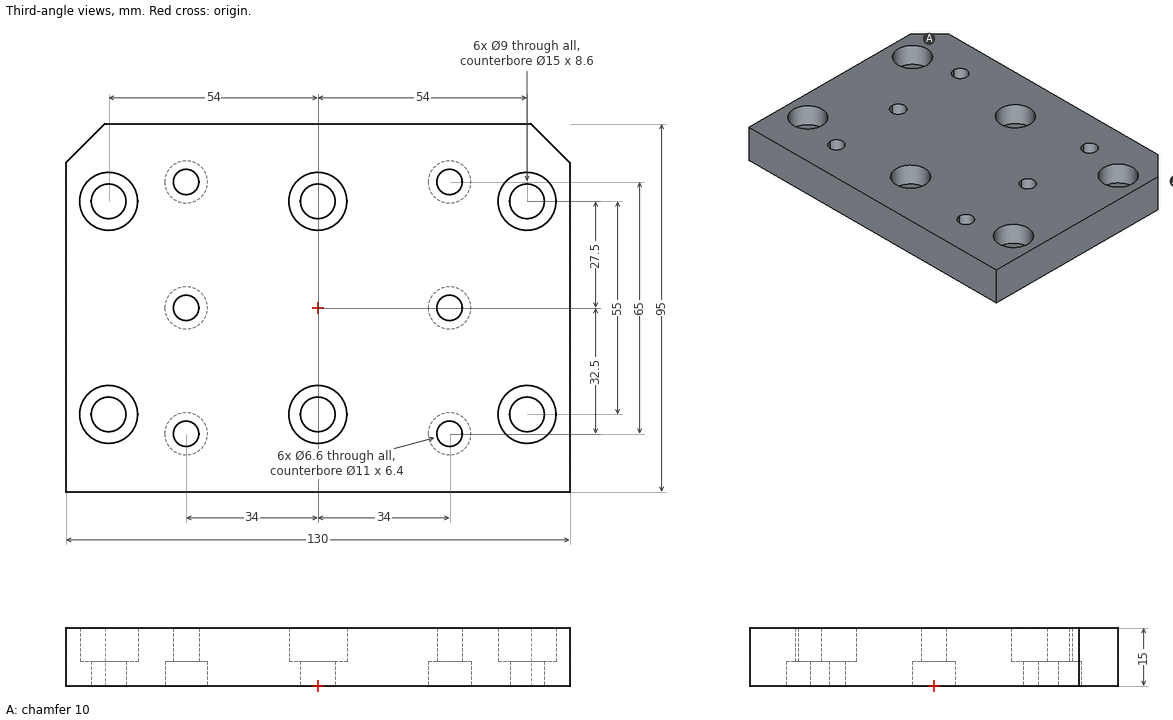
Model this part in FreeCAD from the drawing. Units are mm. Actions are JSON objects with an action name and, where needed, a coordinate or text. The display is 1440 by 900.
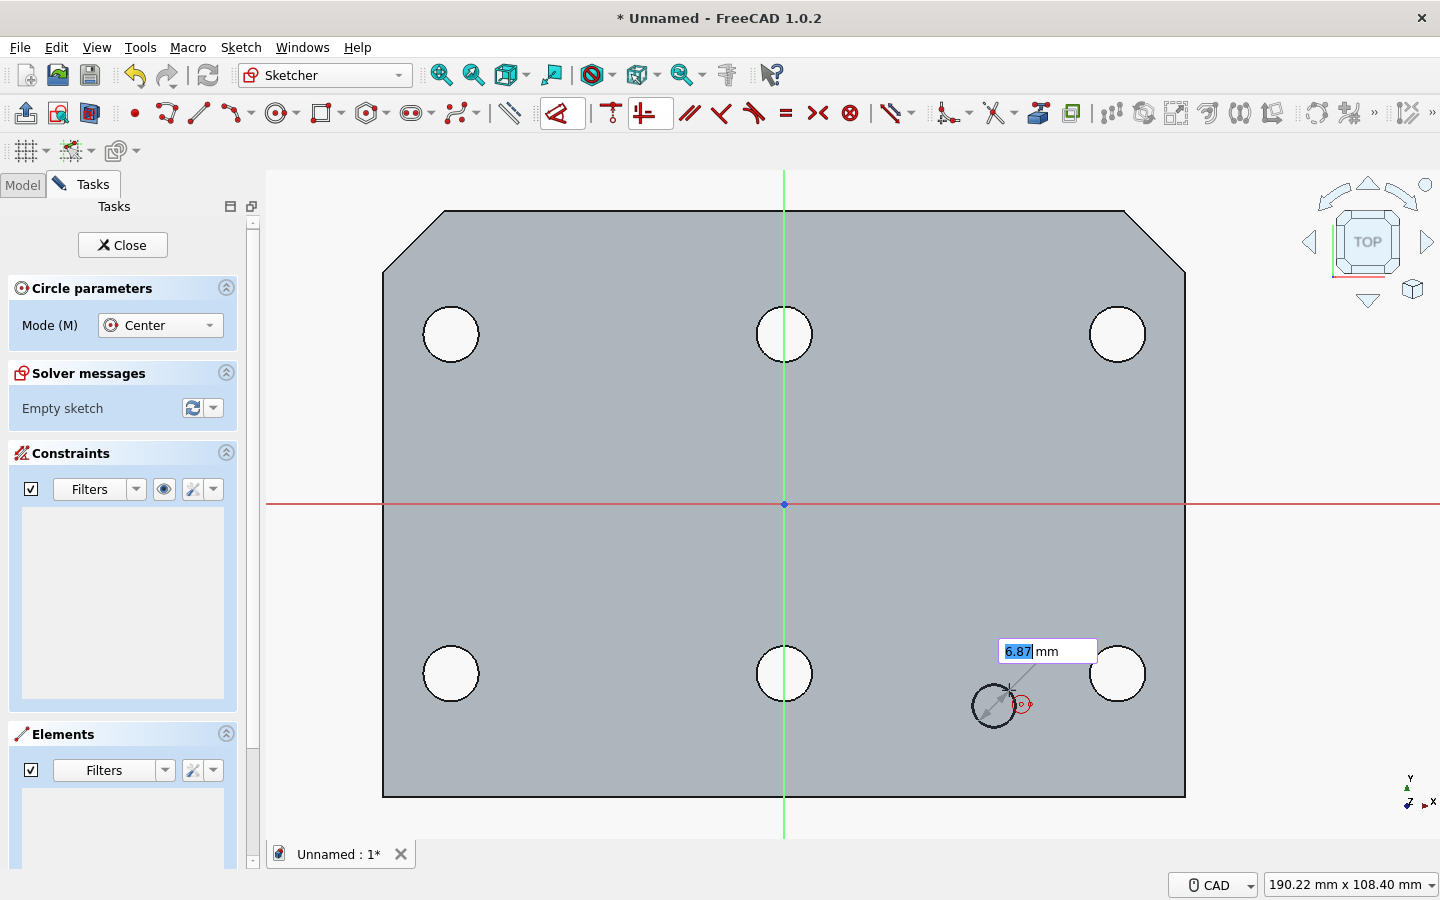
{"action": "type", "text": "6.6"}
{"action": "key", "text": "Return"}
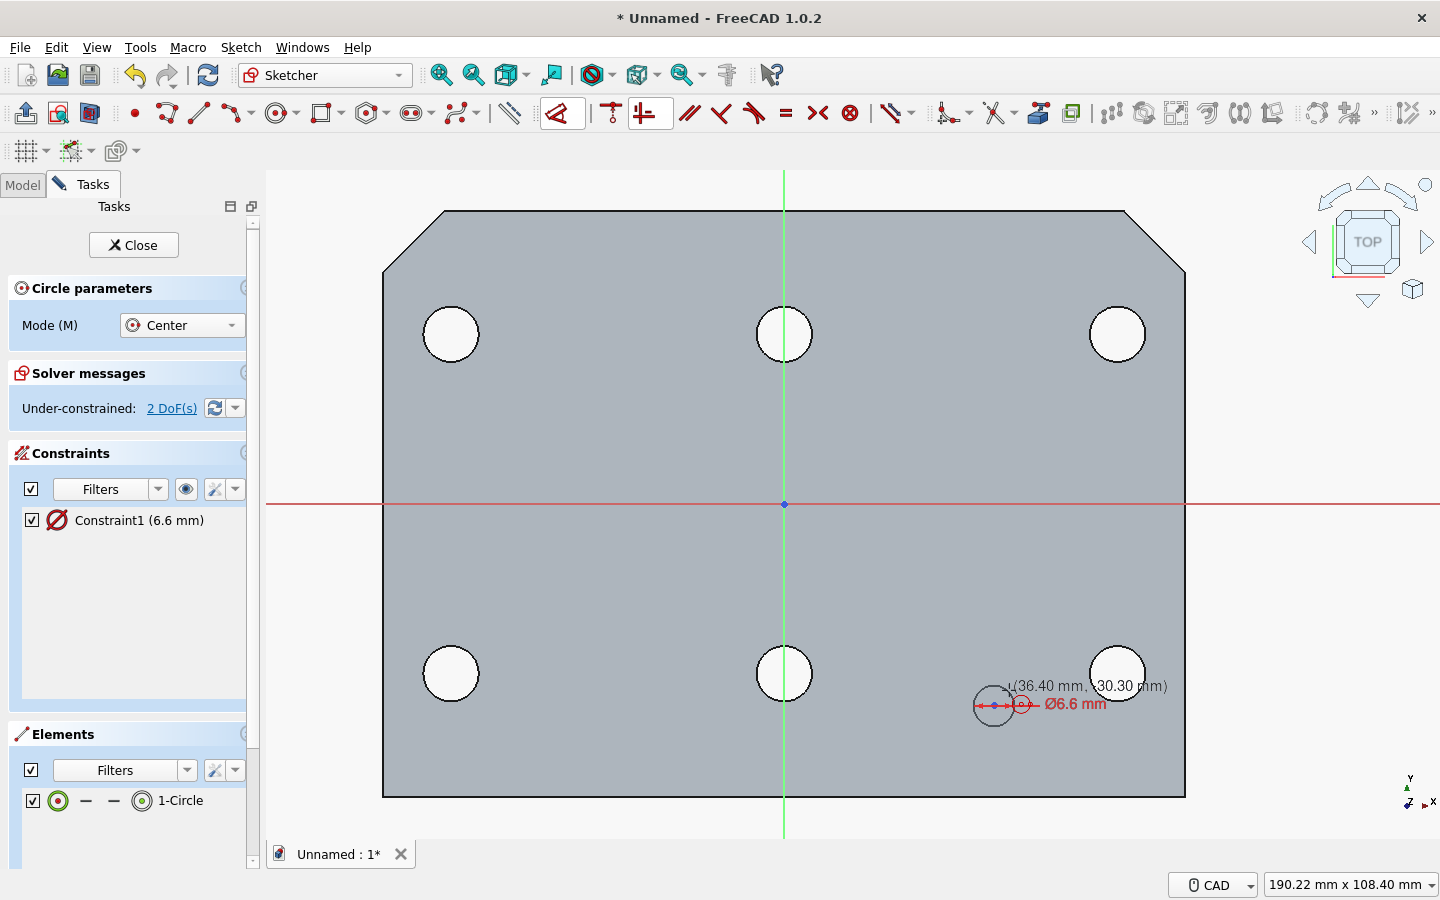
{"action": "left_click", "coordinate": [994, 504]}
{"action": "mouse_move", "coordinate": [1009, 490]}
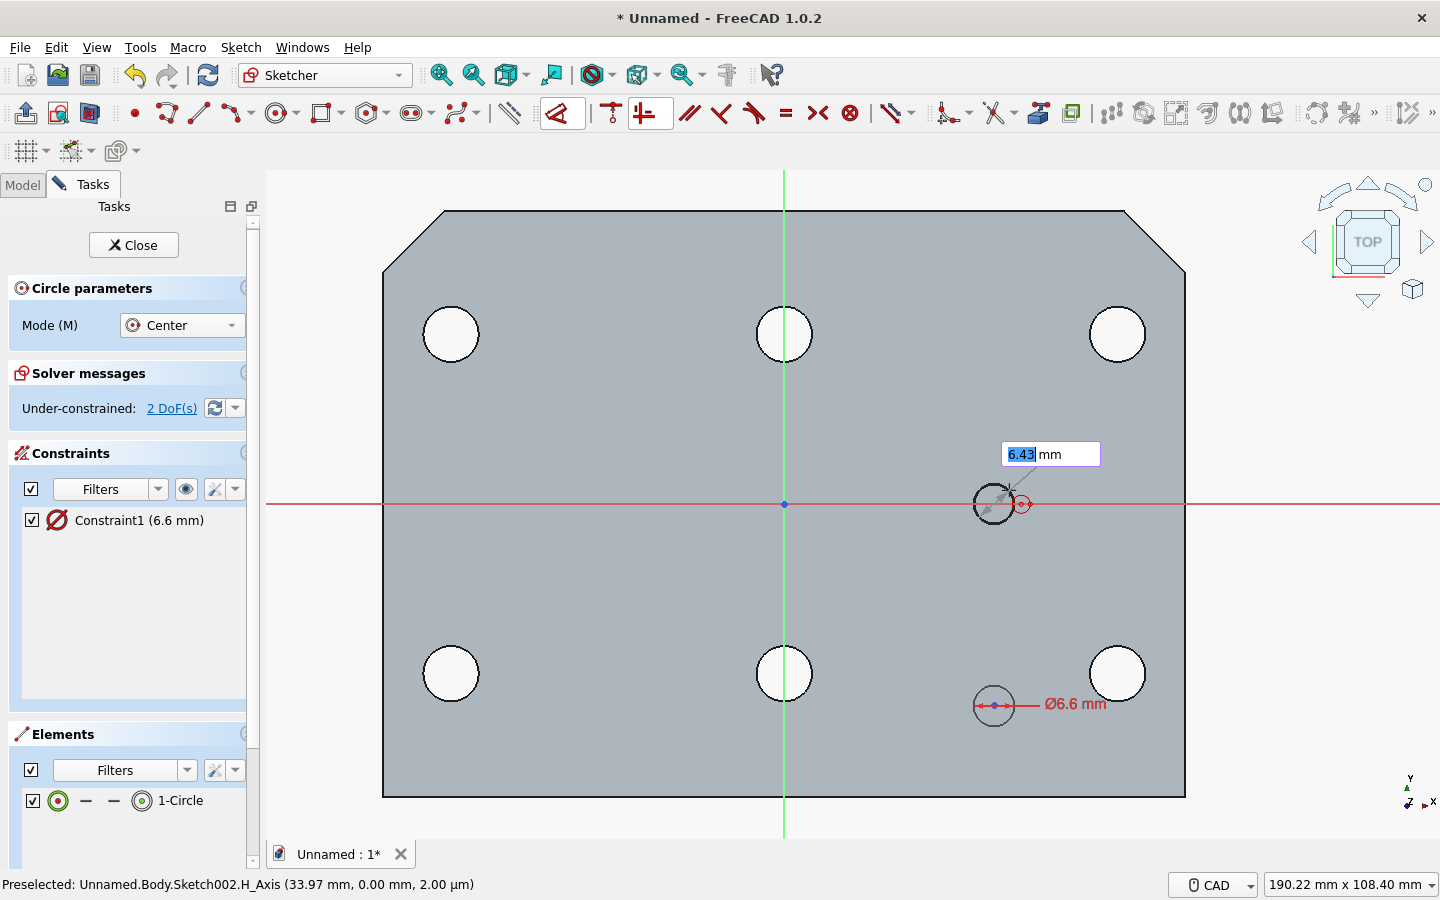
{"action": "type", "text": "6.6"}
{"action": "key", "text": "Return"}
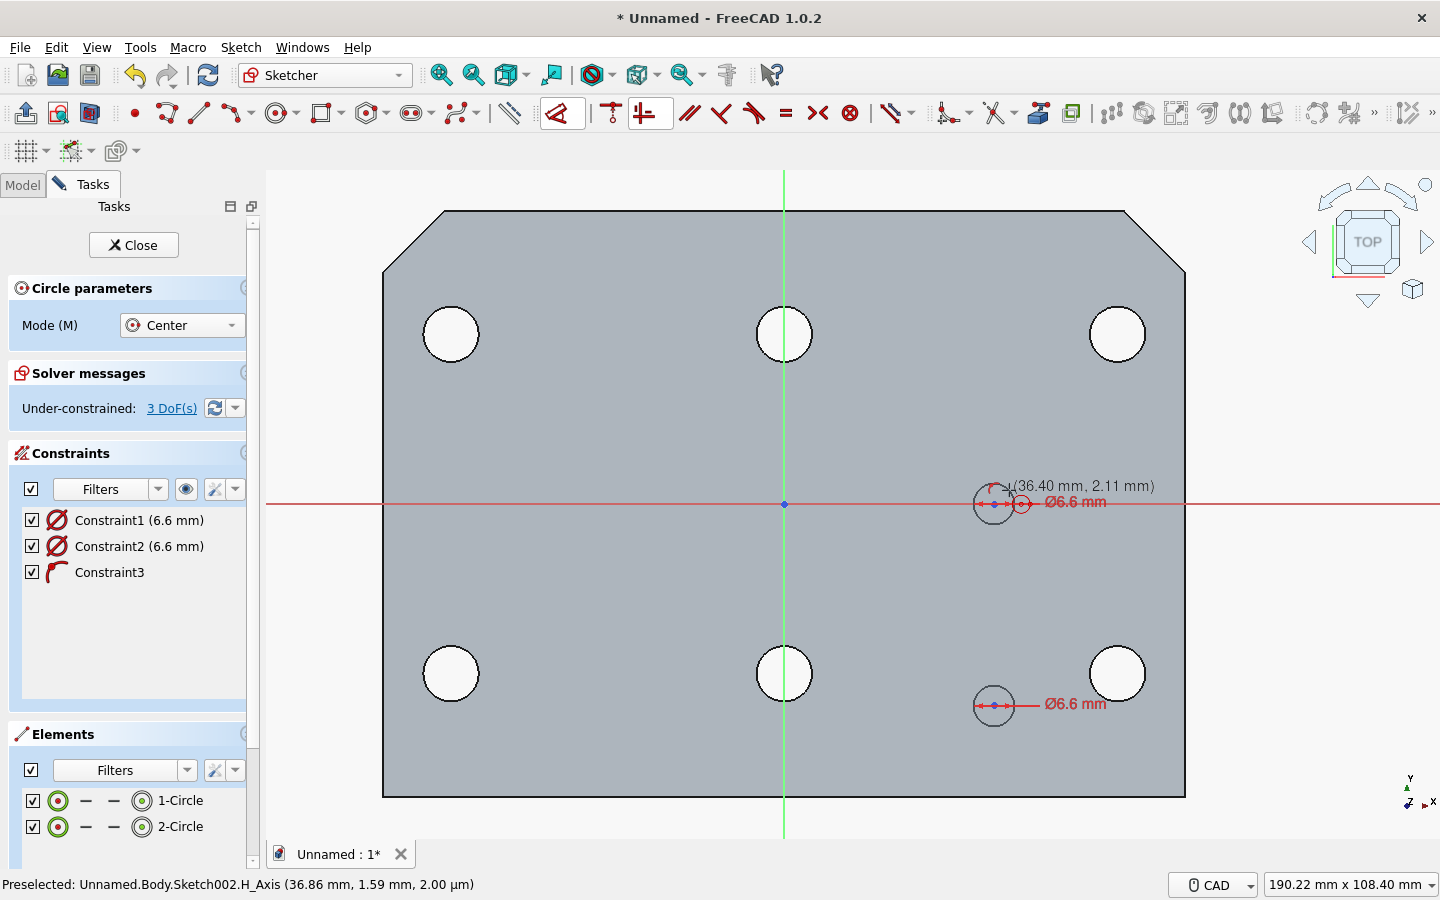
{"action": "left_click", "coordinate": [994, 303]}
{"action": "mouse_move", "coordinate": [1009, 289]}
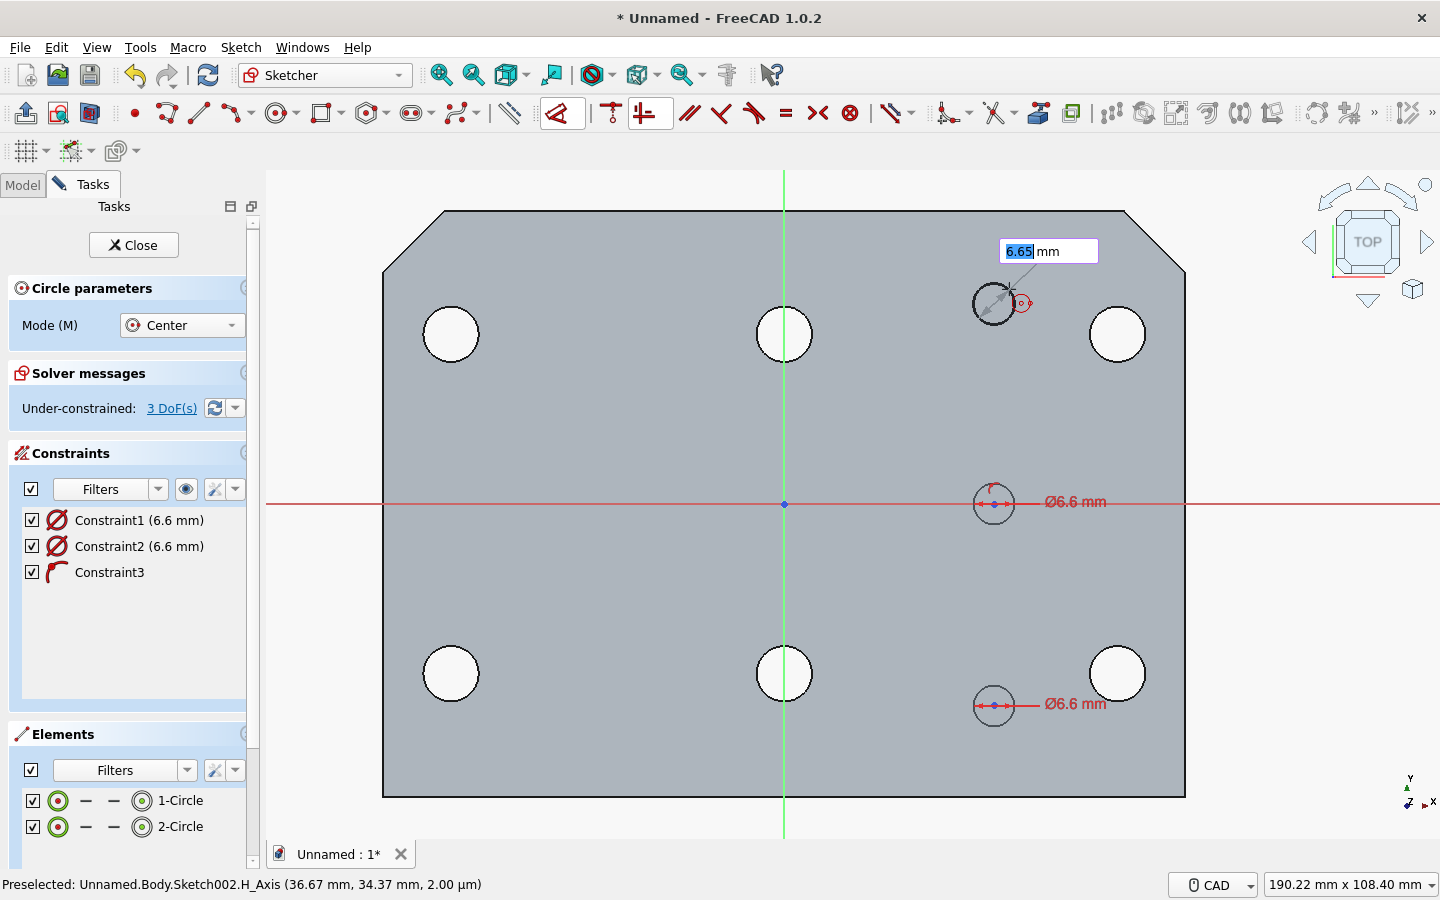
{"action": "type", "text": "6.6"}
{"action": "key", "text": "Return"}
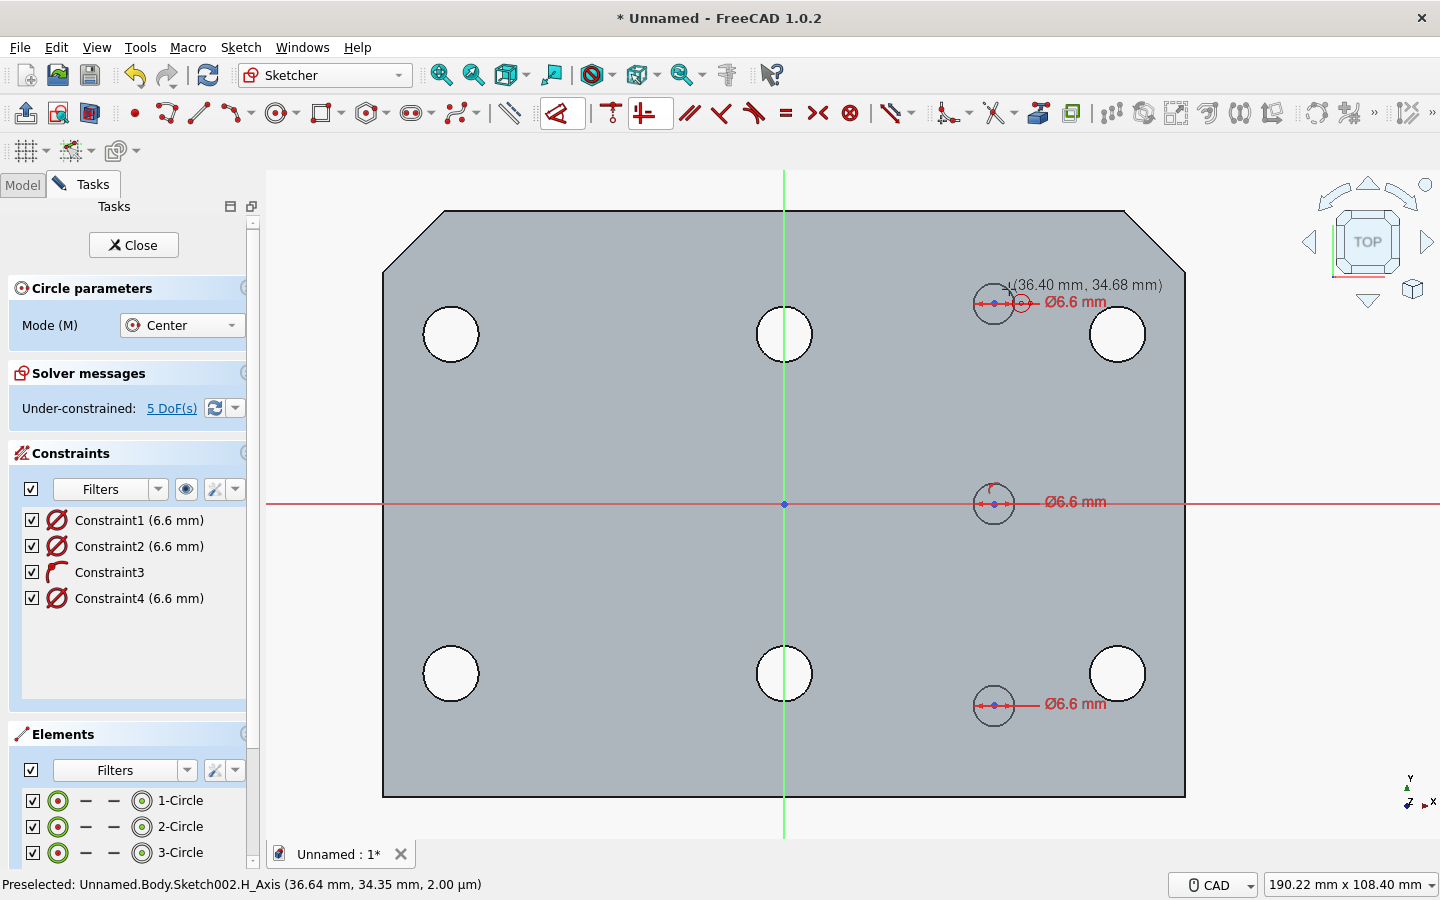
{"action": "left_click", "coordinate": [574, 705]}
{"action": "mouse_move", "coordinate": [589, 690]}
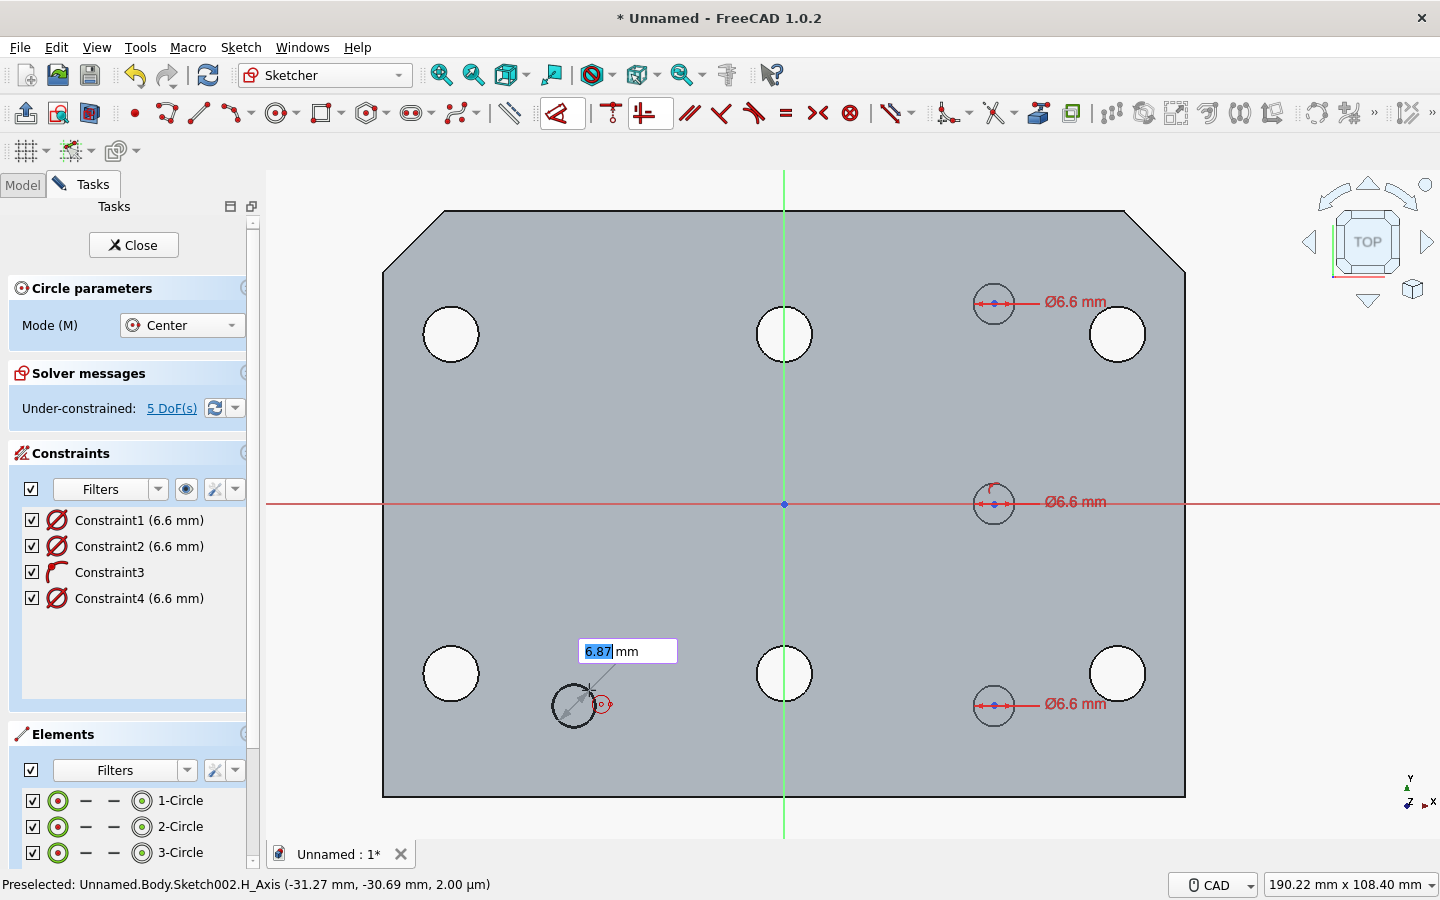
{"action": "type", "text": "6.6"}
{"action": "key", "text": "Return"}